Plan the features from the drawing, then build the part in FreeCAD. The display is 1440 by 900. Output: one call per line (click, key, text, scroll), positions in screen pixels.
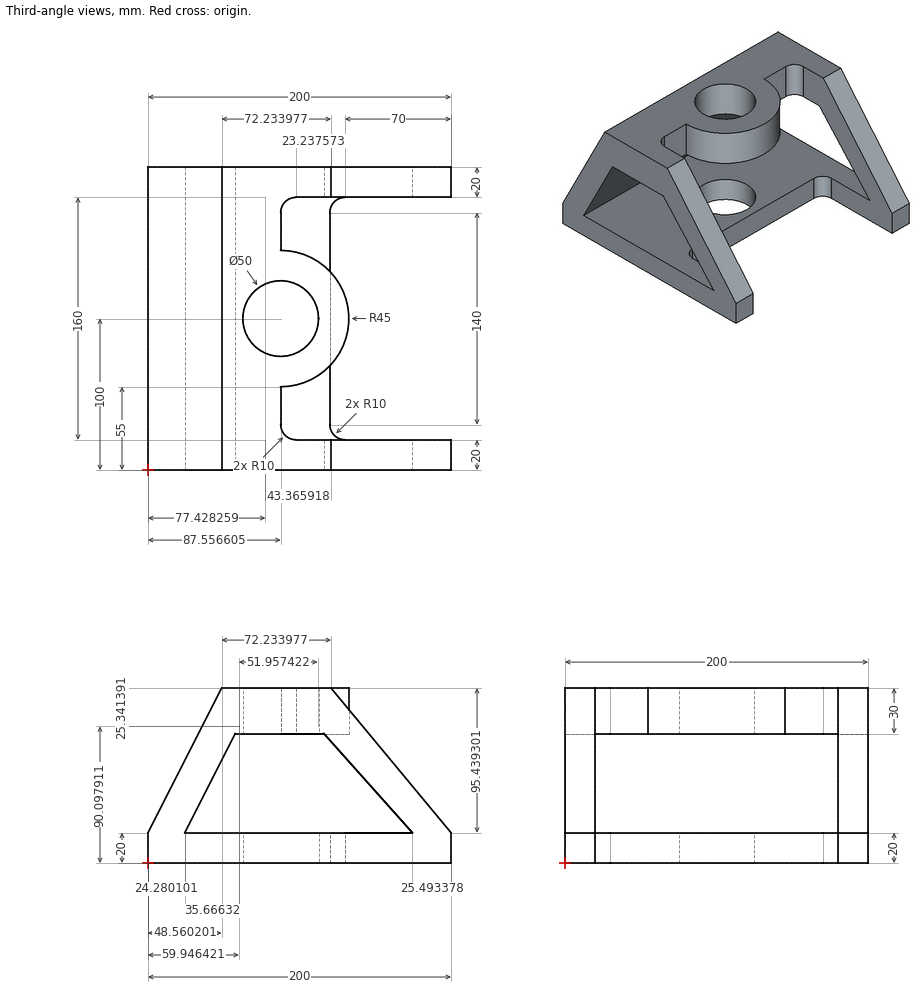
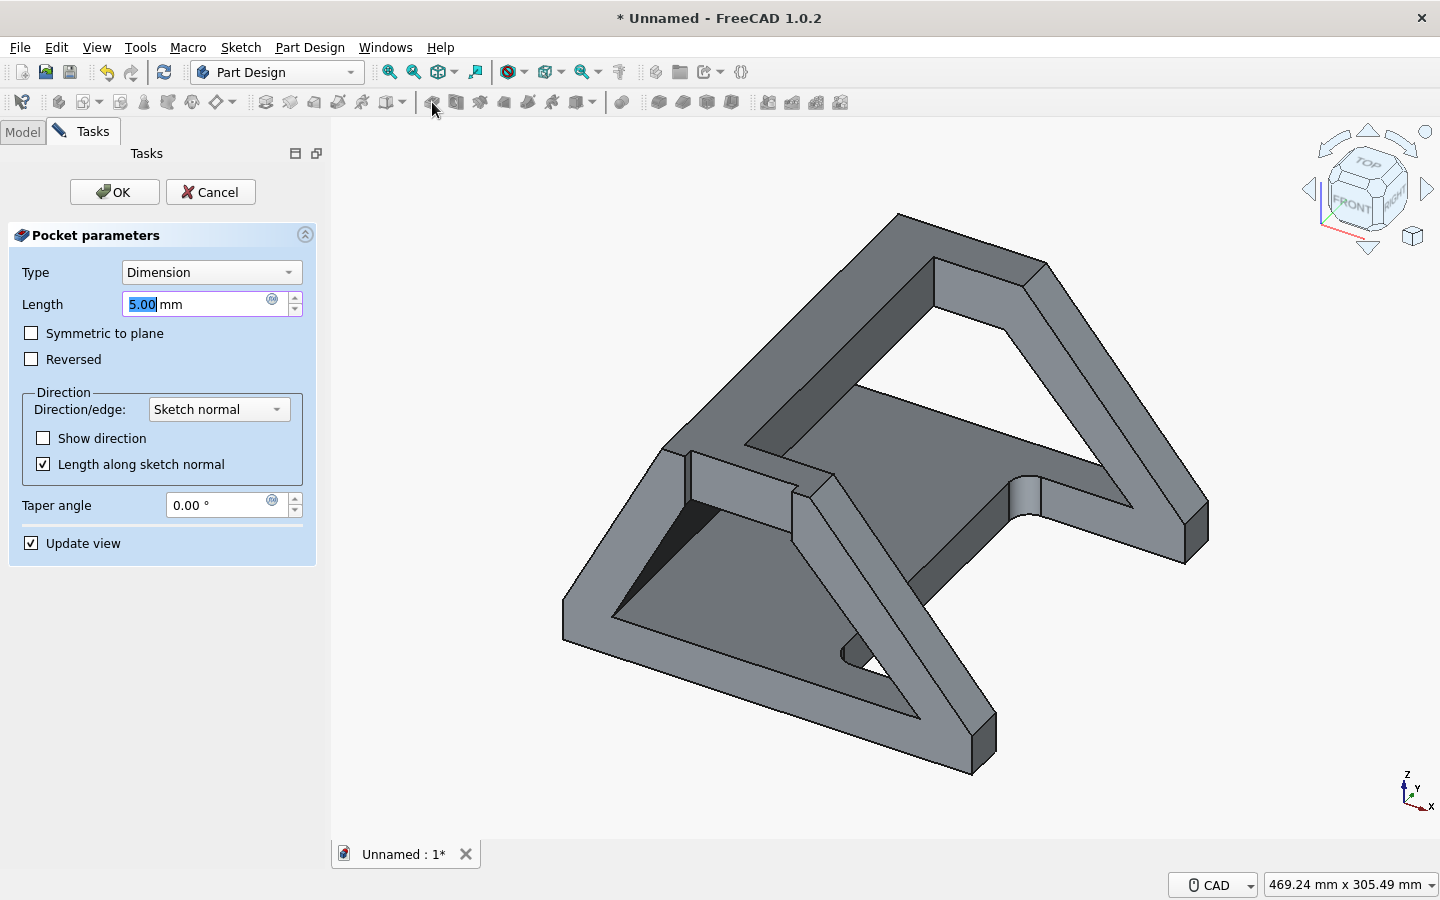
text(200)
key(Tab)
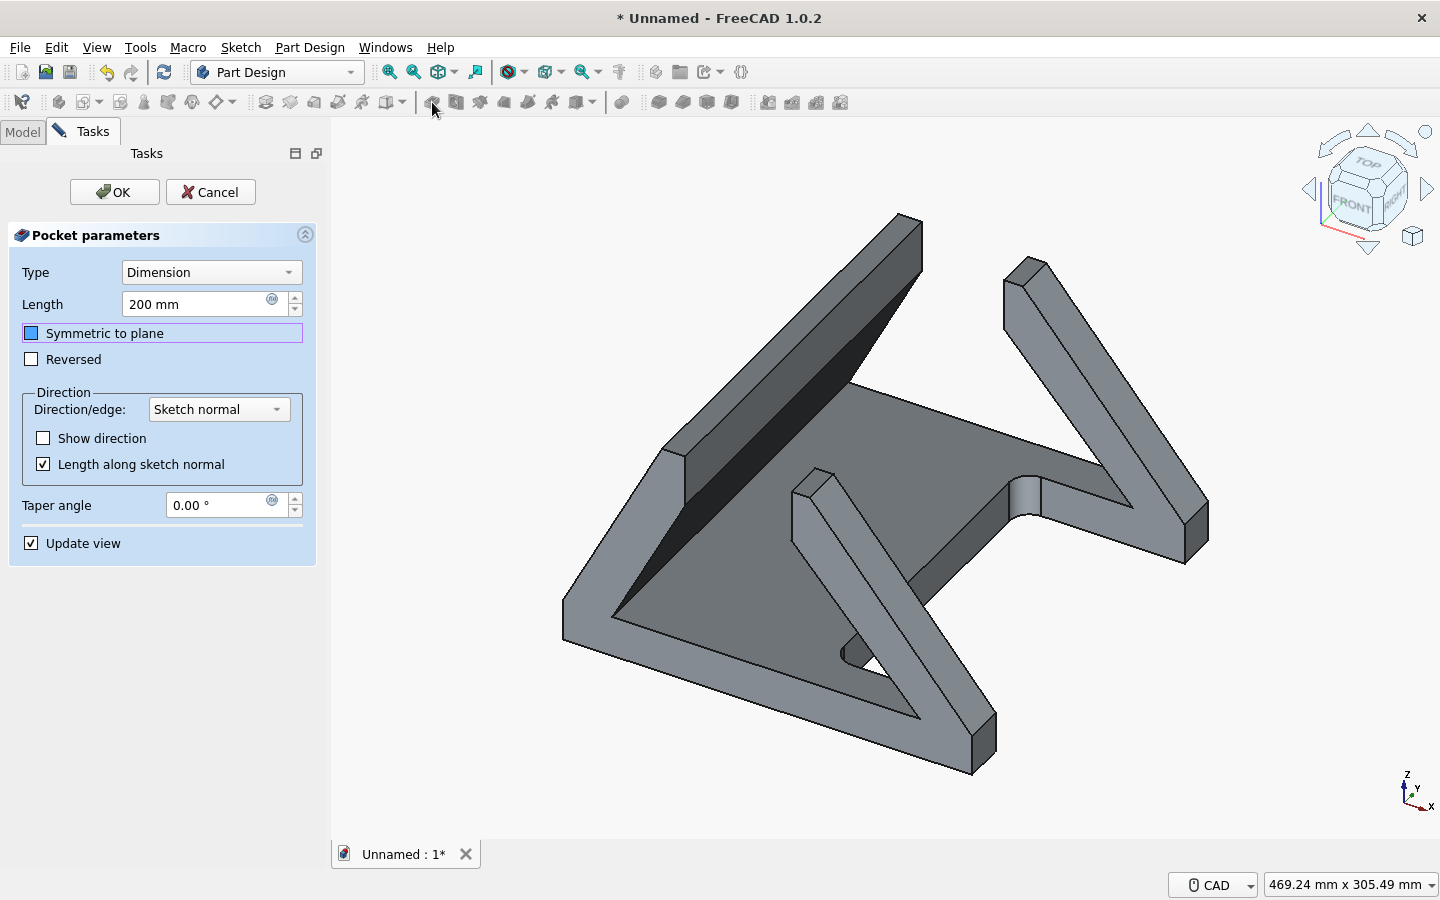
click(115, 192)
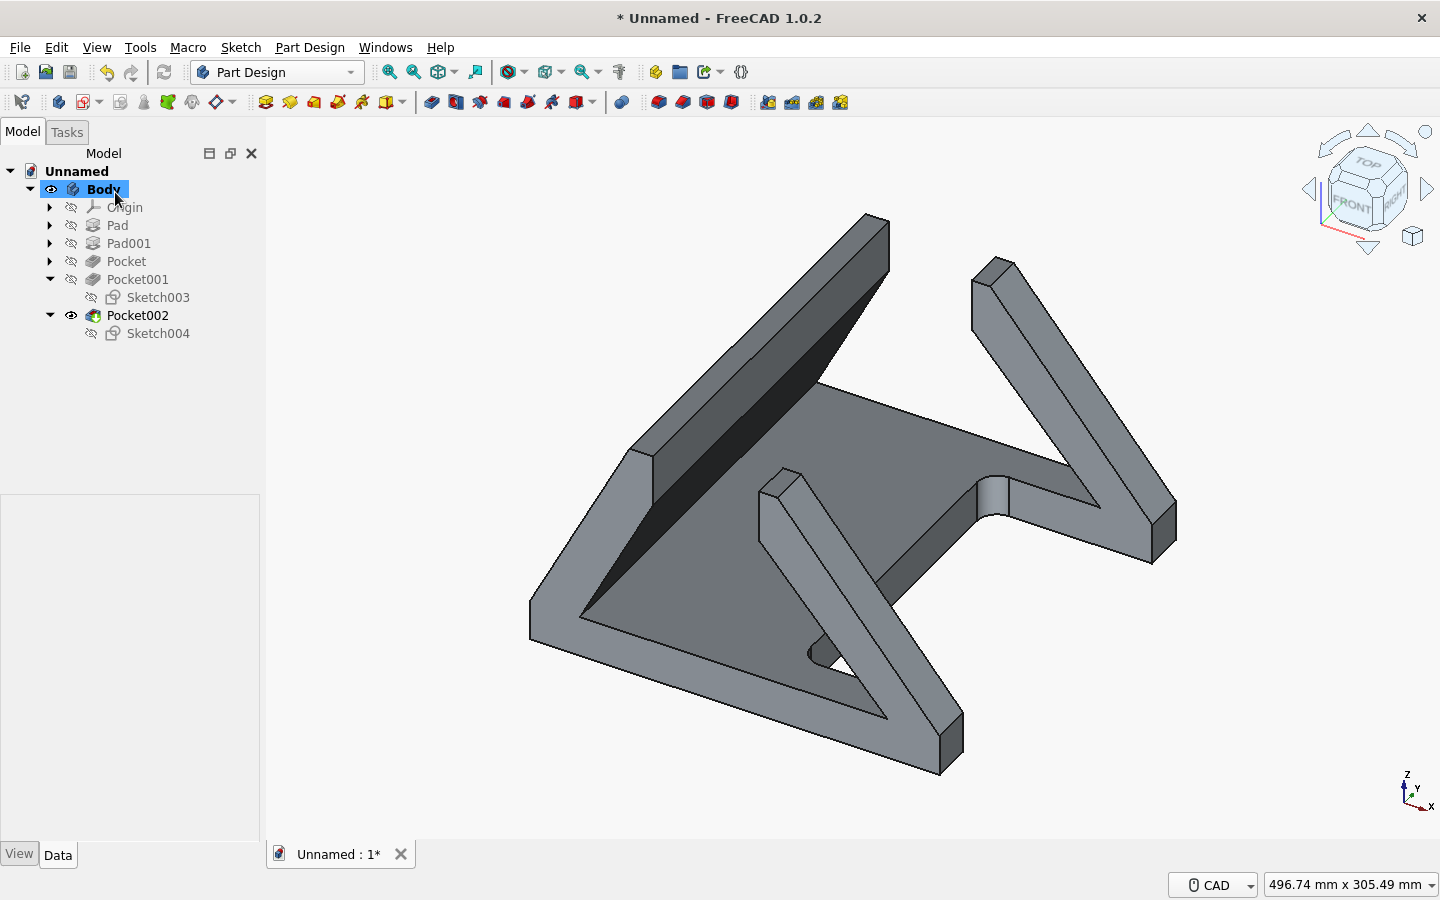
click(861, 234)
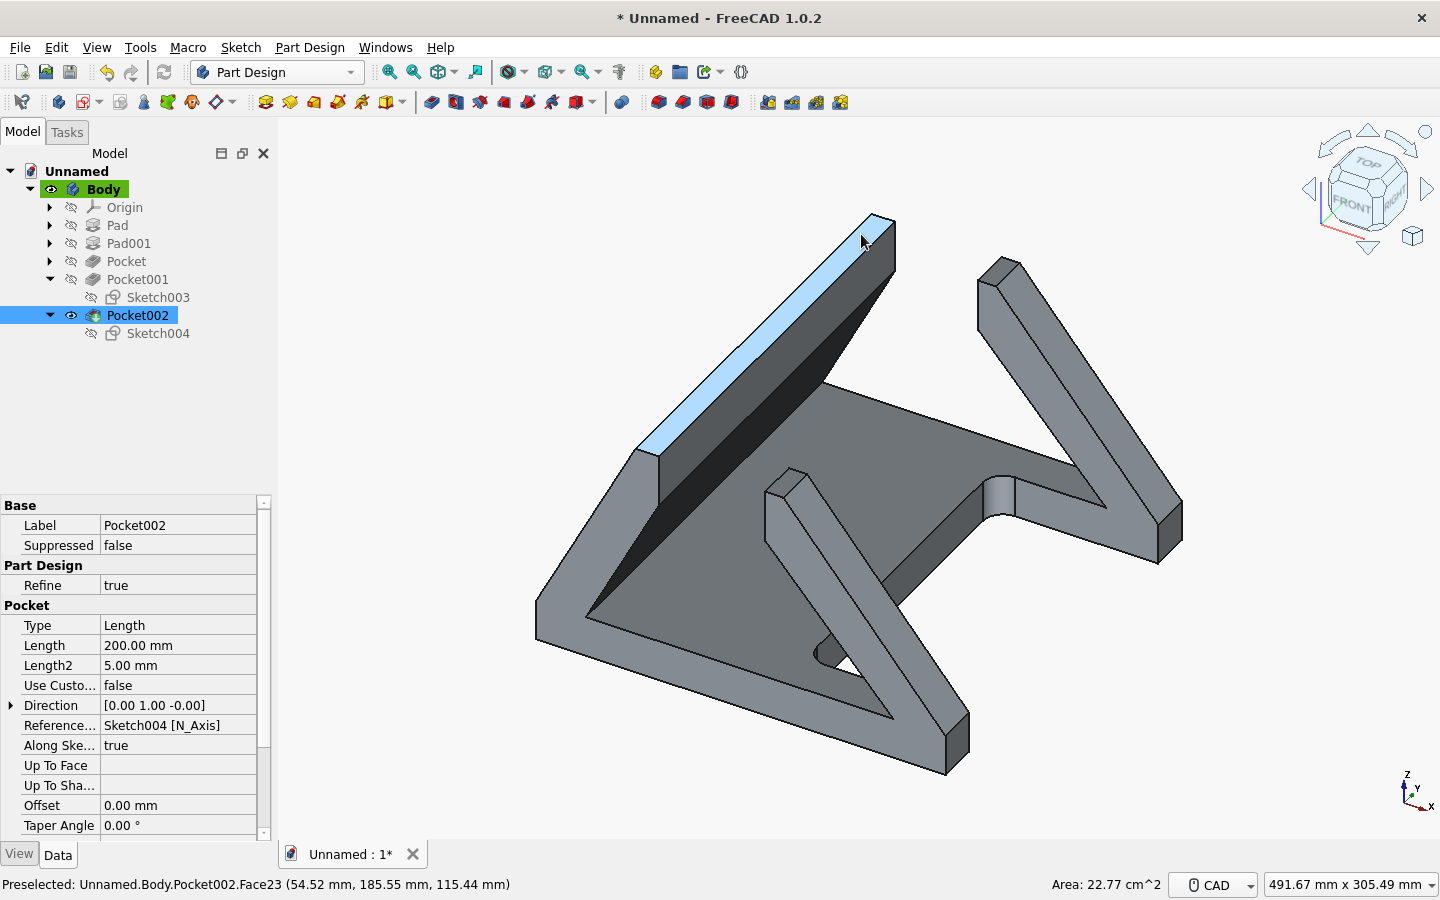
click(84, 102)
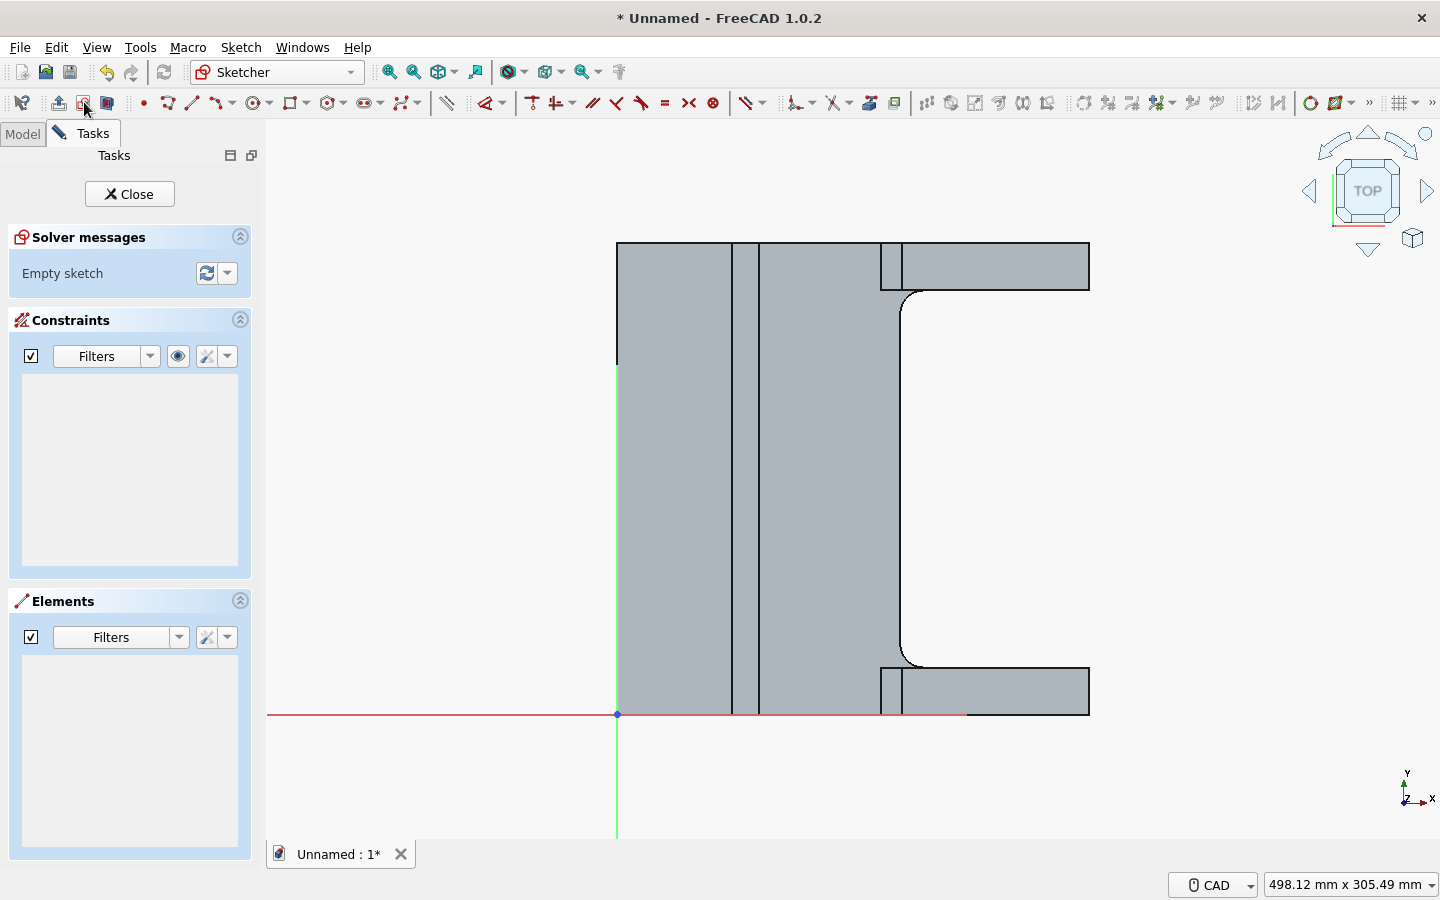
click(192, 104)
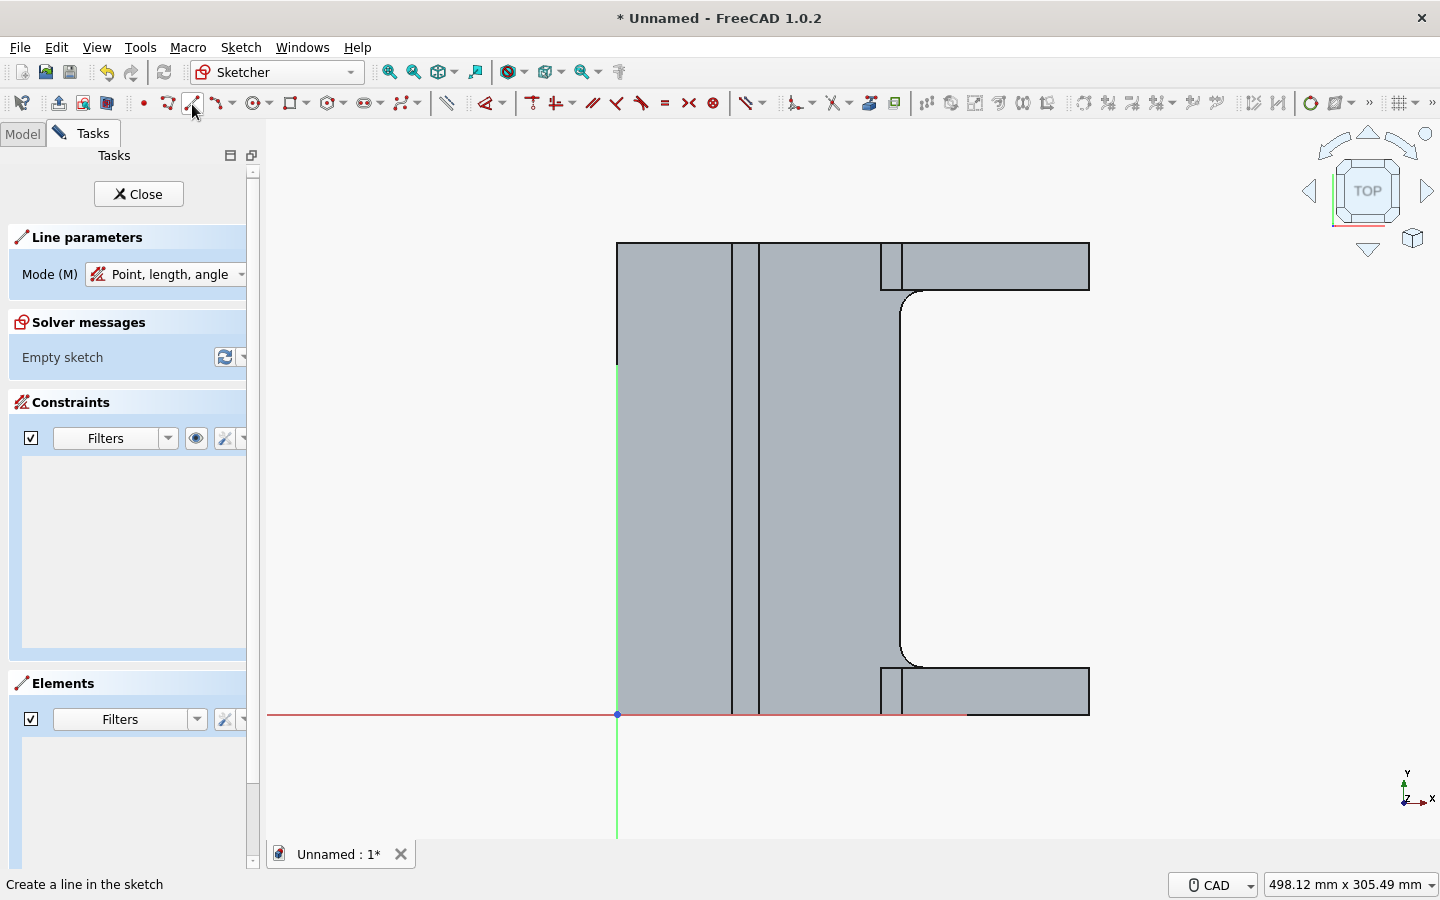
click(824, 644)
click(824, 314)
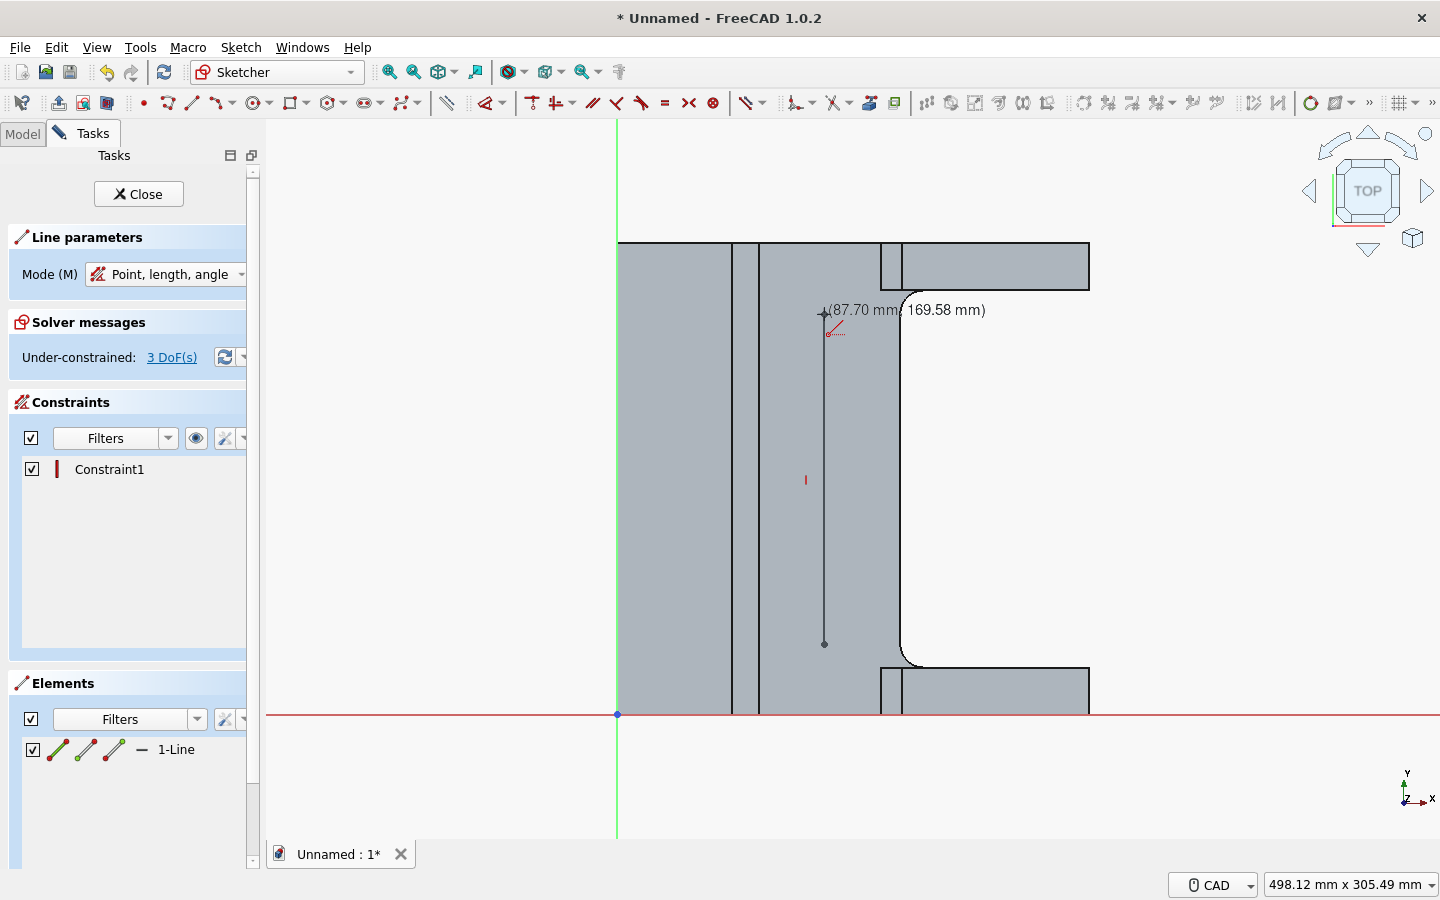
click(168, 104)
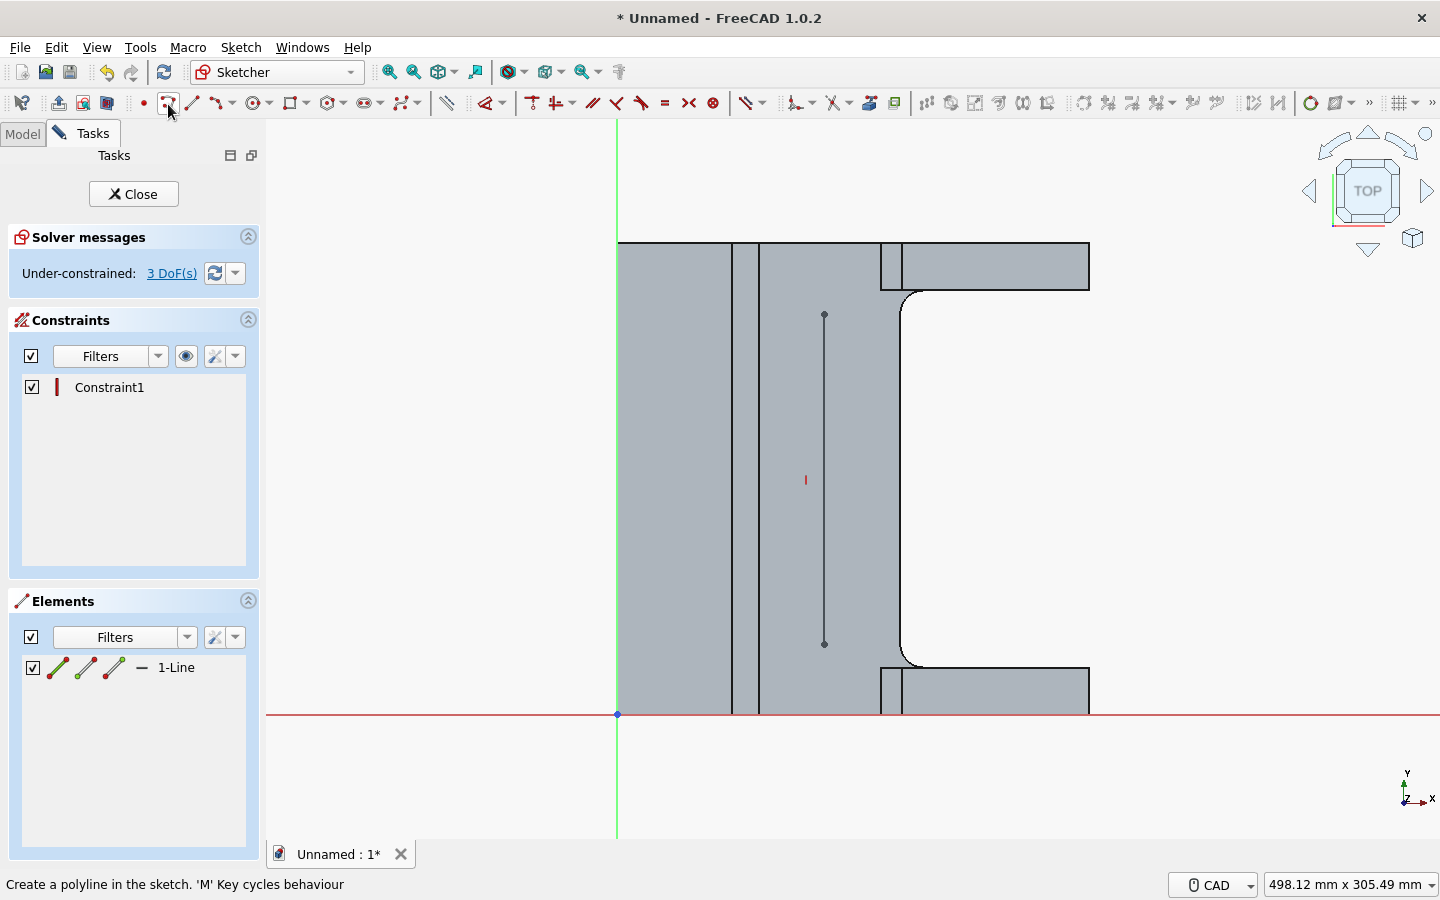
click(847, 290)
click(902, 290)
click(902, 243)
click(732, 243)
click(732, 715)
click(902, 706)
click(902, 668)
click(847, 668)
right_click(847, 668)